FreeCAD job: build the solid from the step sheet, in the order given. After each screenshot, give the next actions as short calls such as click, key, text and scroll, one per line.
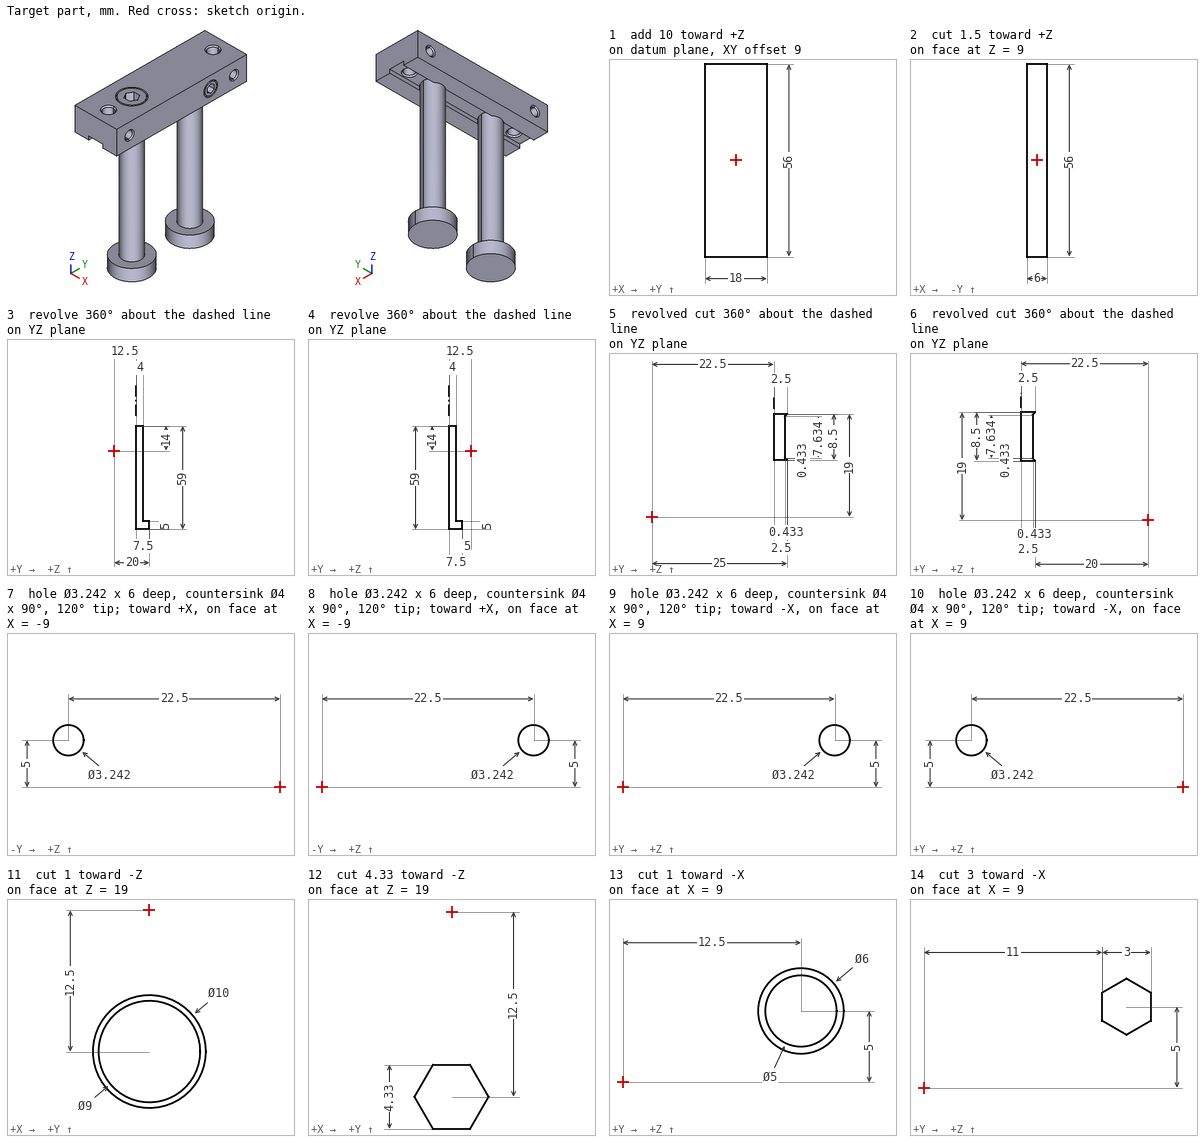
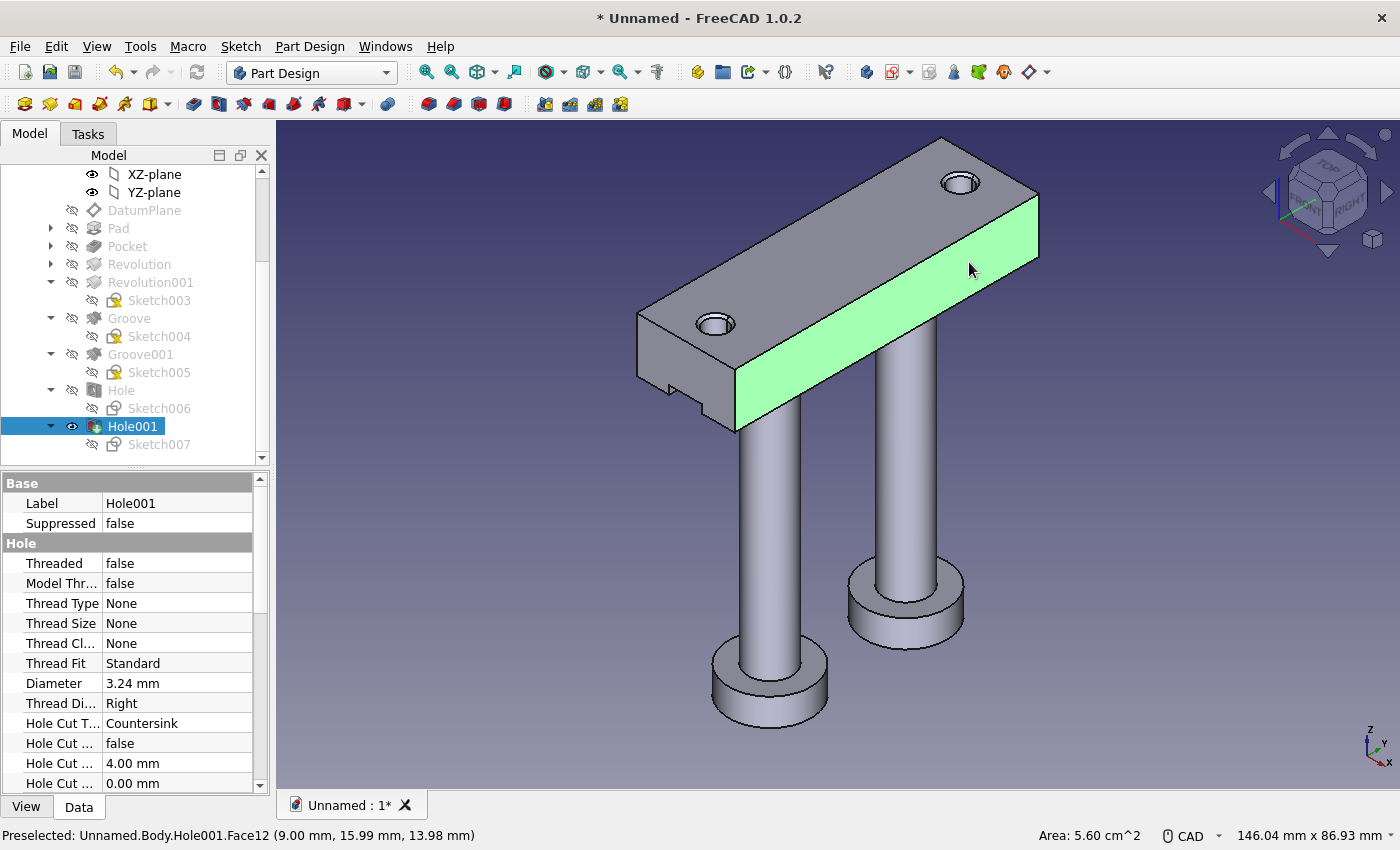
click(892, 72)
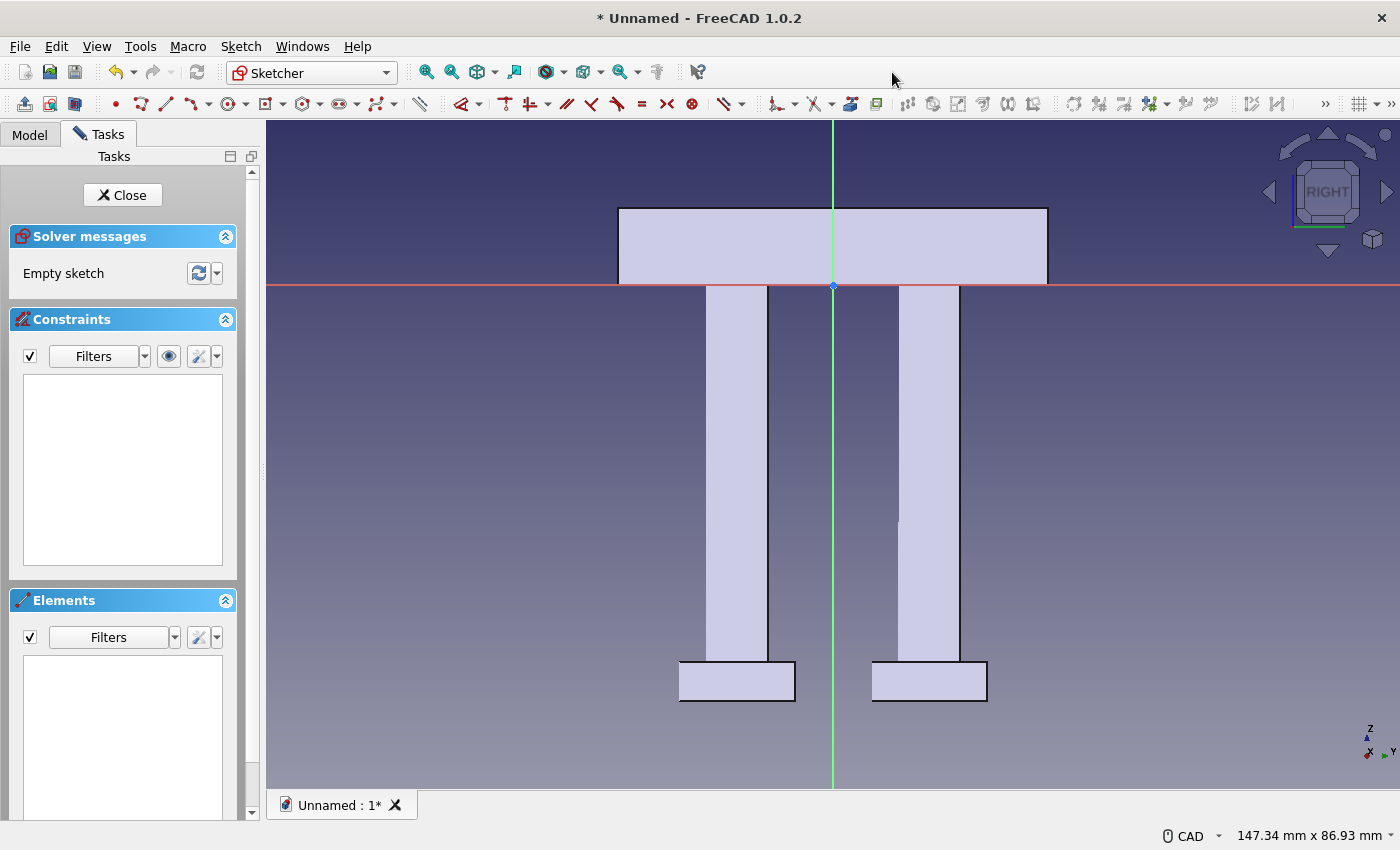
scroll(1022, 233, up, 14)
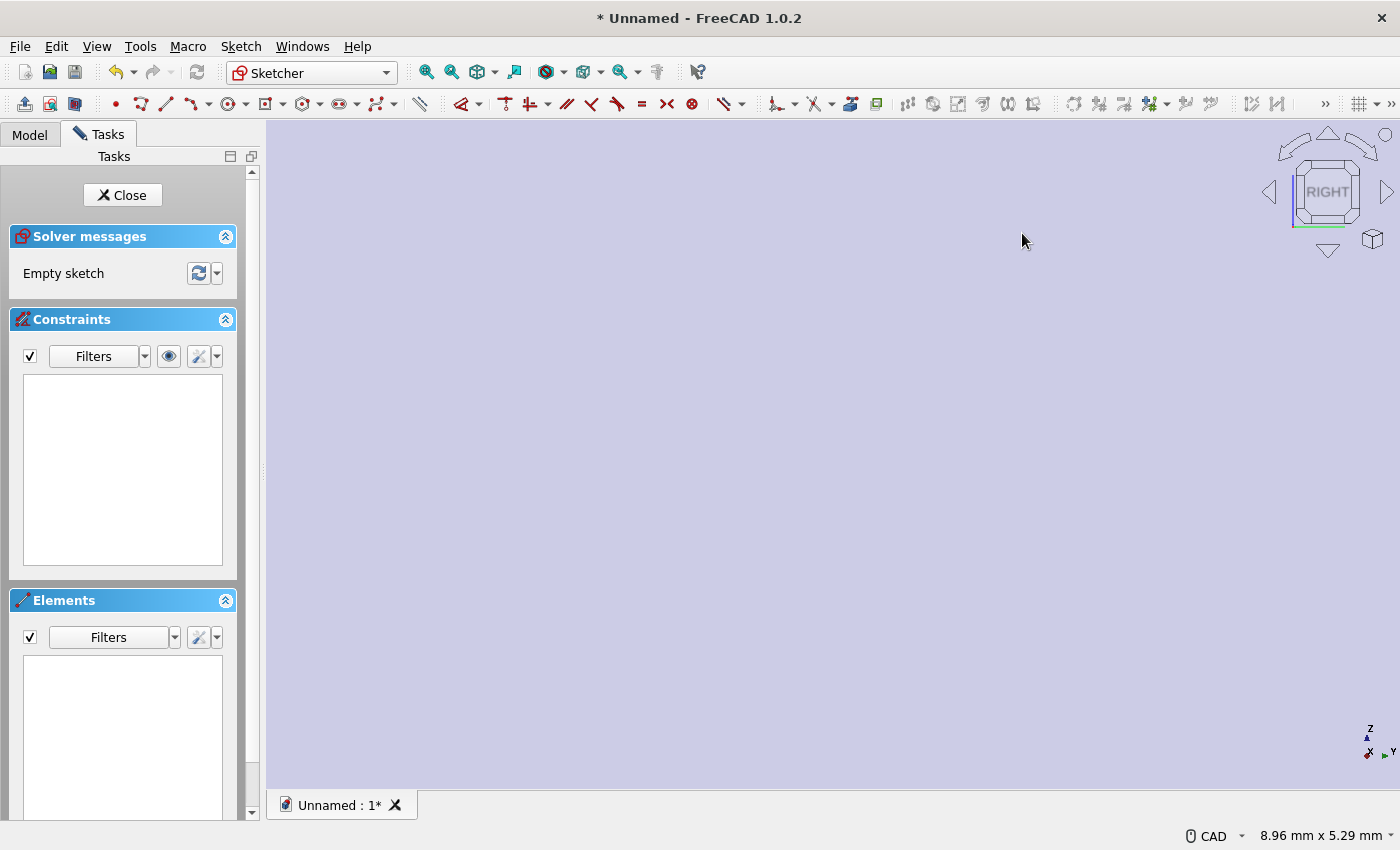
click(228, 104)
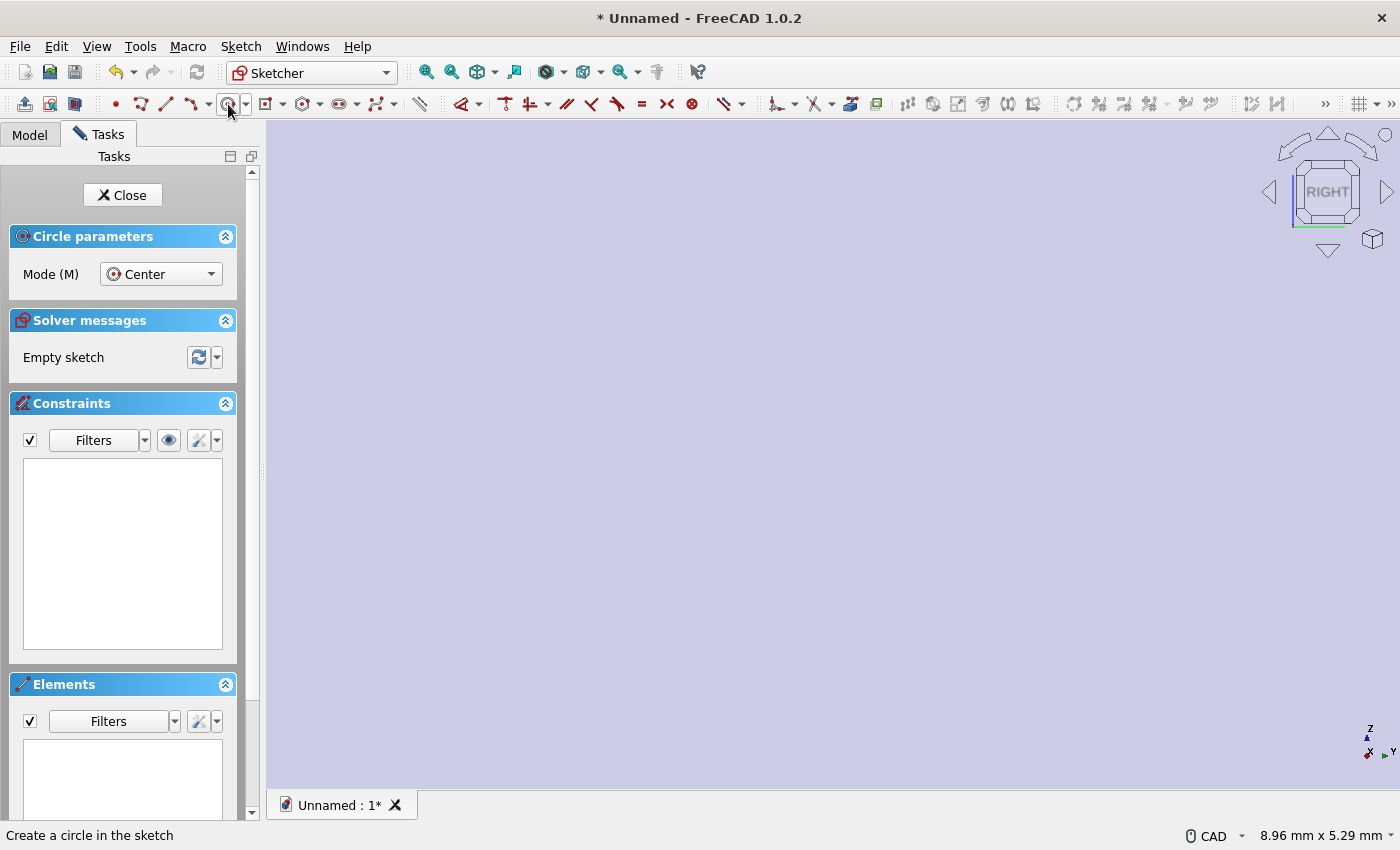
click(751, 456)
move(896, 311)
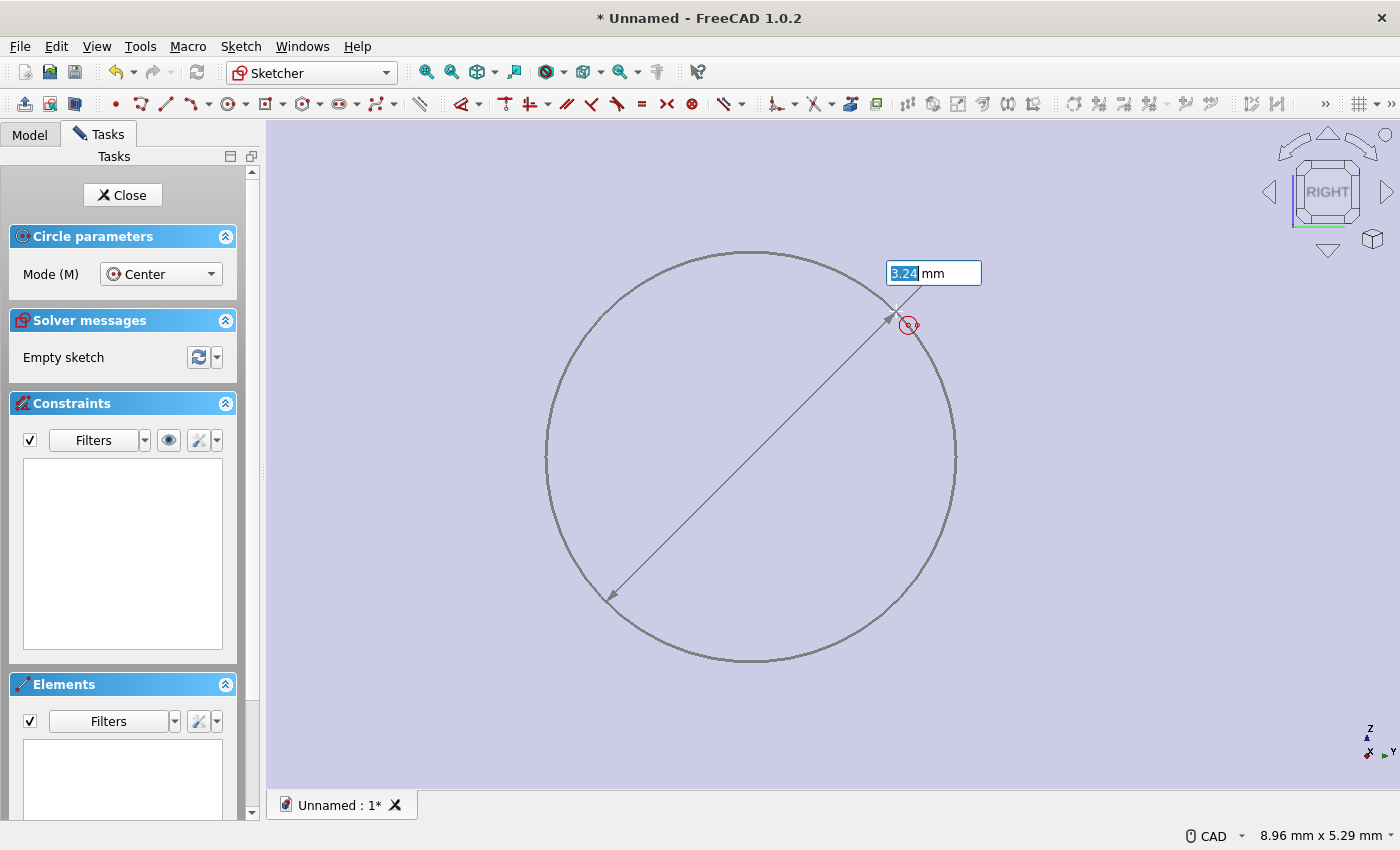
text(3.242)
key(Return)
key(Escape)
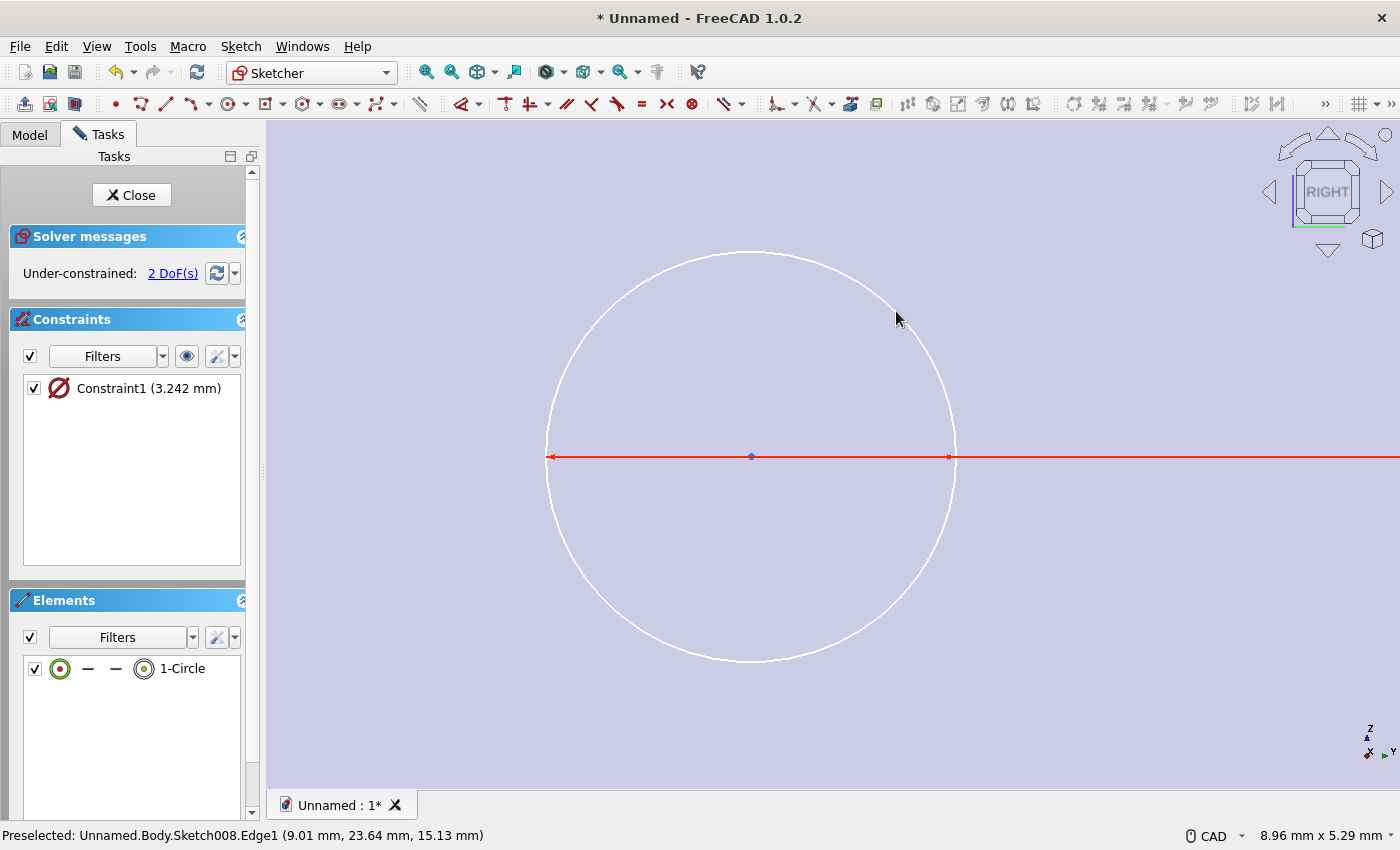
click(460, 104)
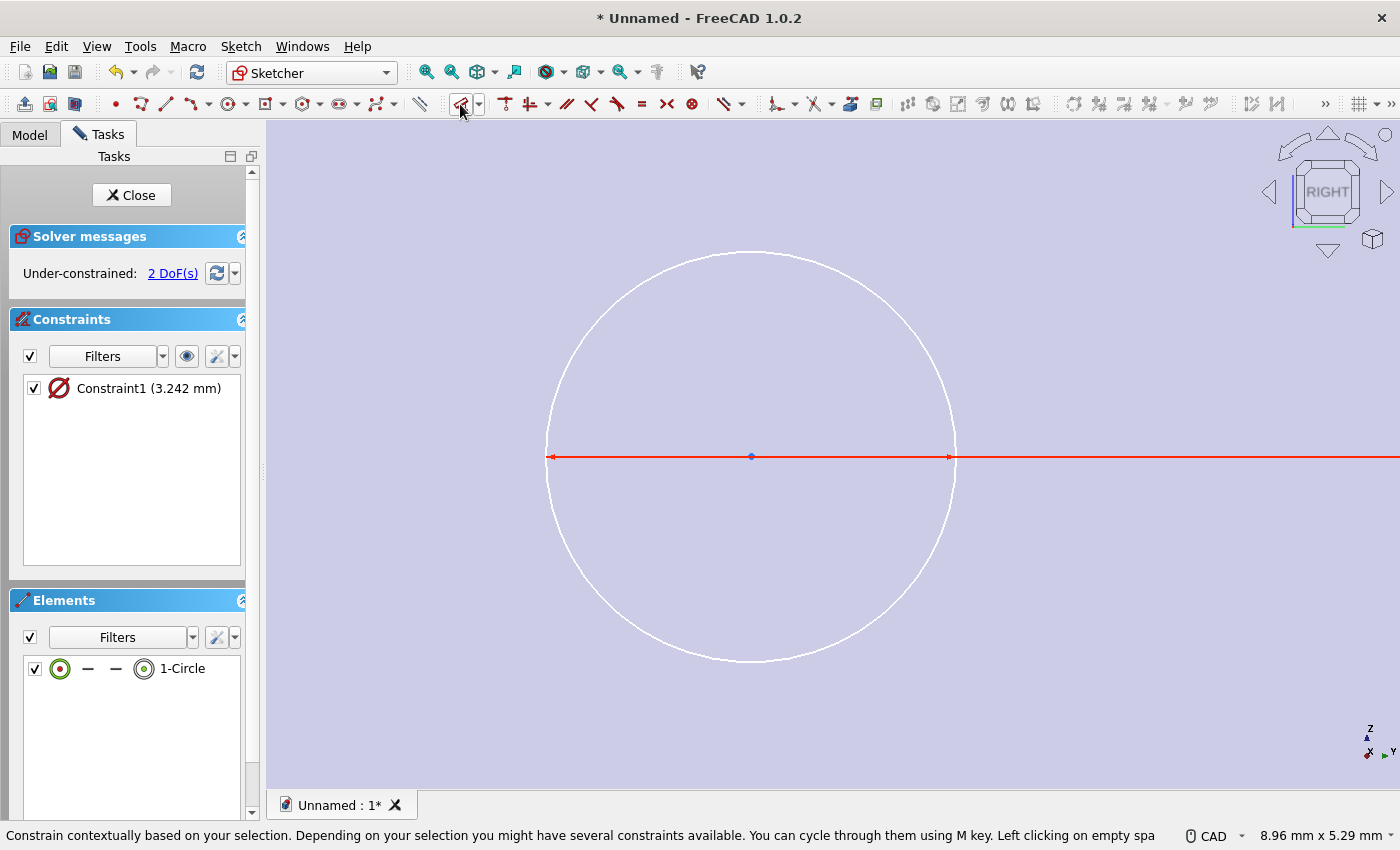
click(751, 457)
click(785, 609)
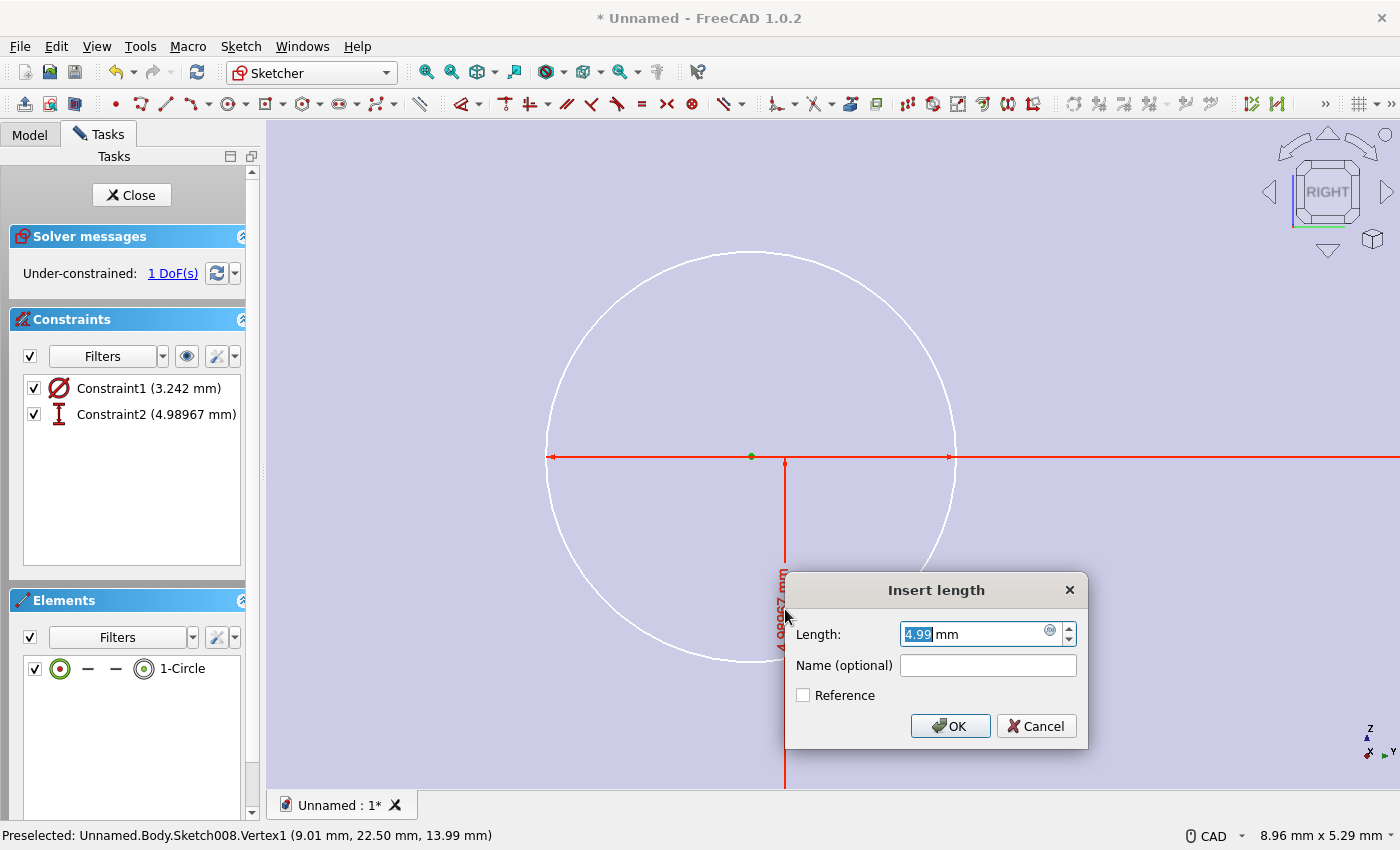
text(5)
key(Return)